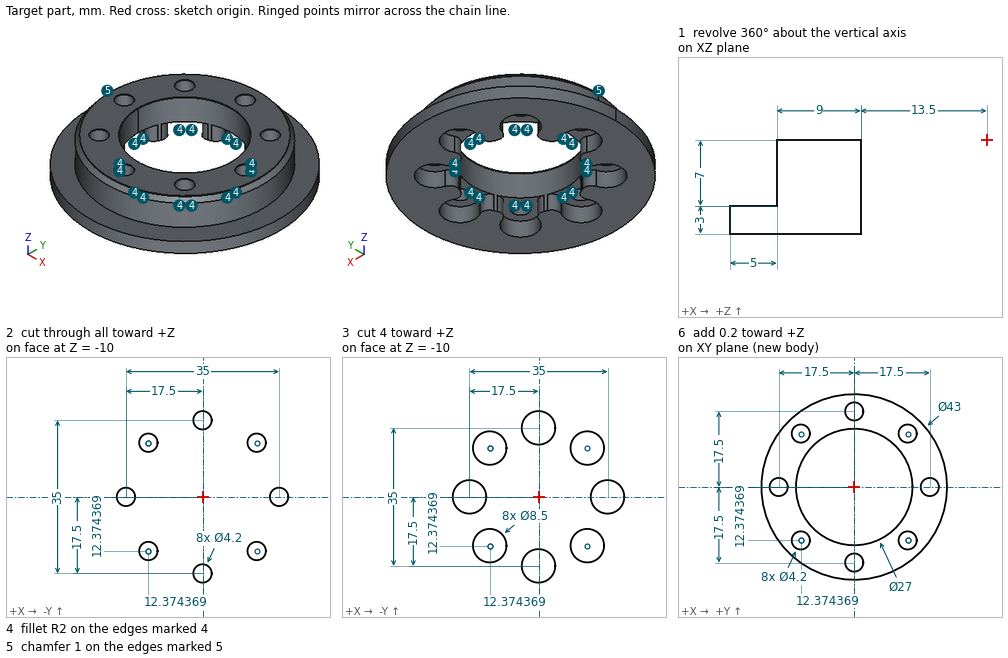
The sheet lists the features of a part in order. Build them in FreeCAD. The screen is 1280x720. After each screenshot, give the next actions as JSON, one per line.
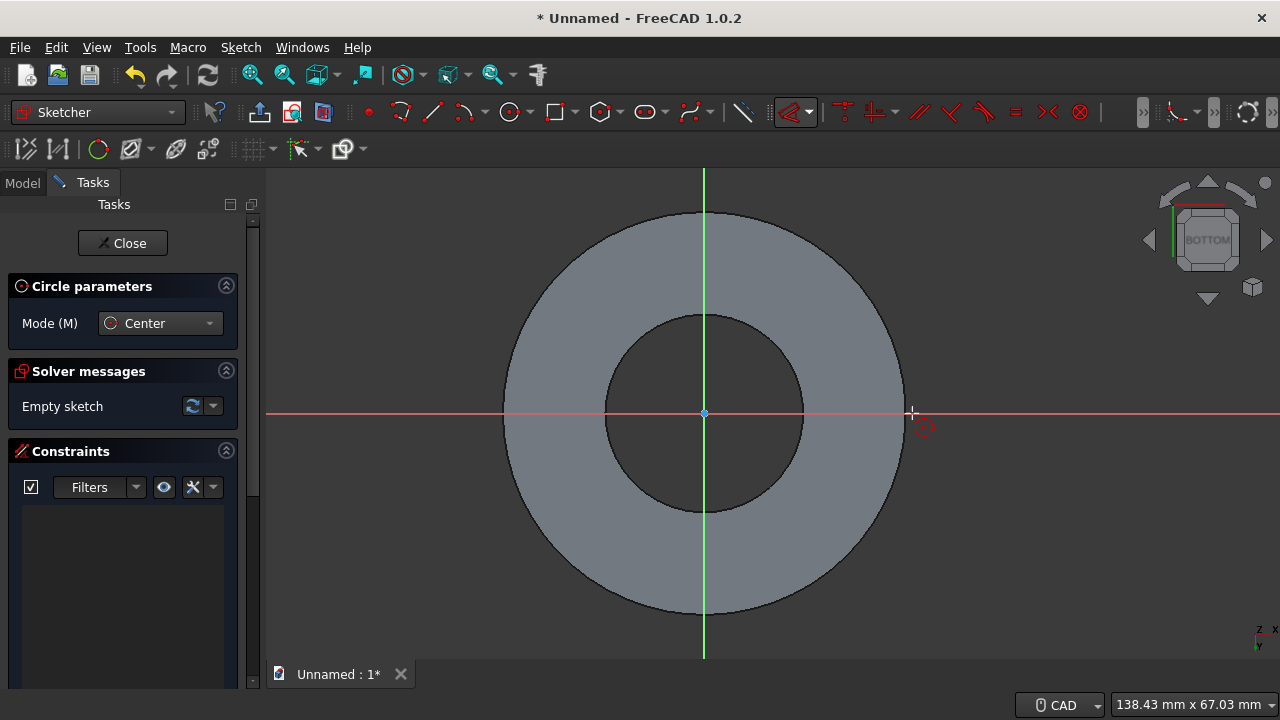
{"action": "scroll", "coordinate": [704, 542], "scroll_direction": "up", "scroll_amount": 2}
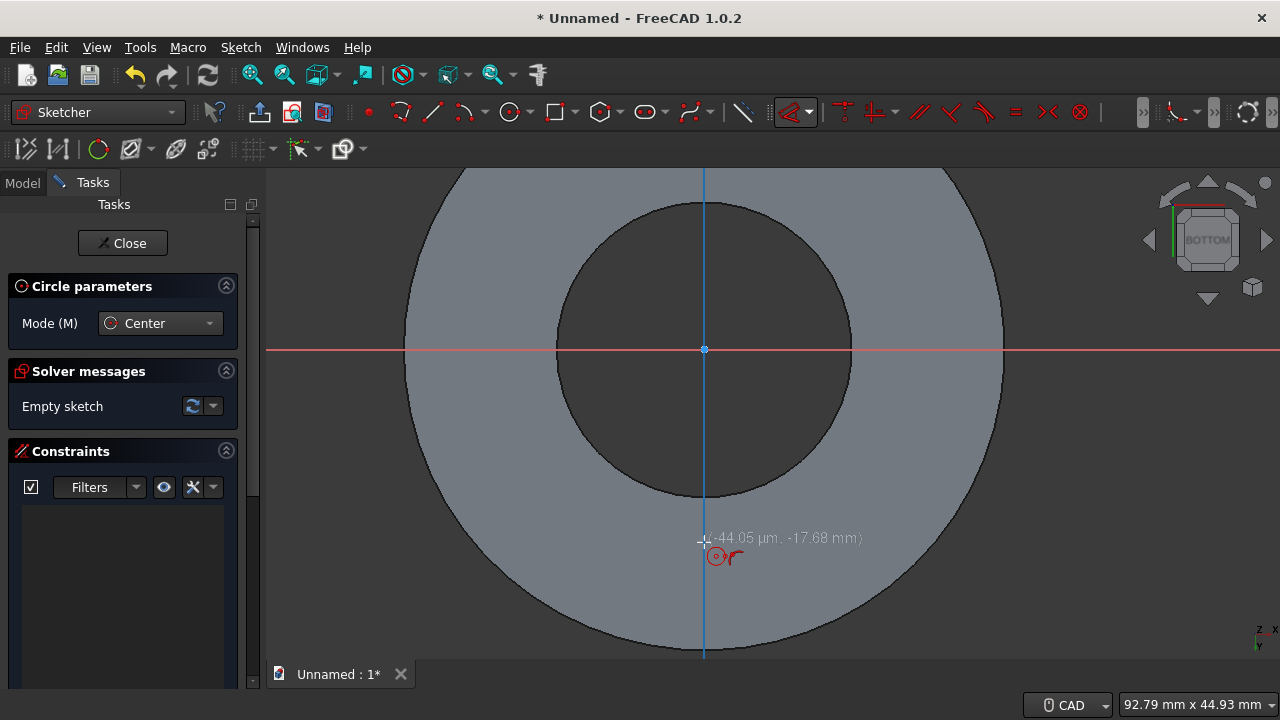
{"action": "left_click", "coordinate": [704, 541]}
{"action": "mouse_move", "coordinate": [720, 525]}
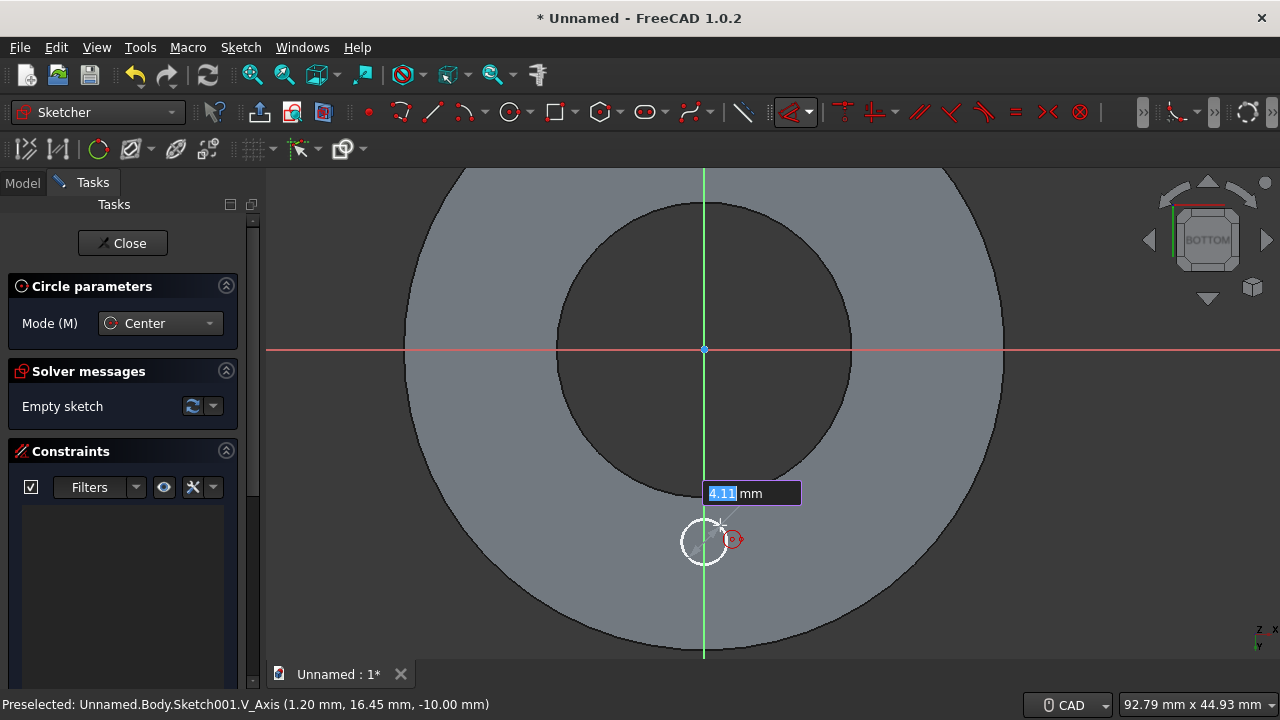
{"action": "type", "text": "4.2"}
{"action": "key", "text": "Return"}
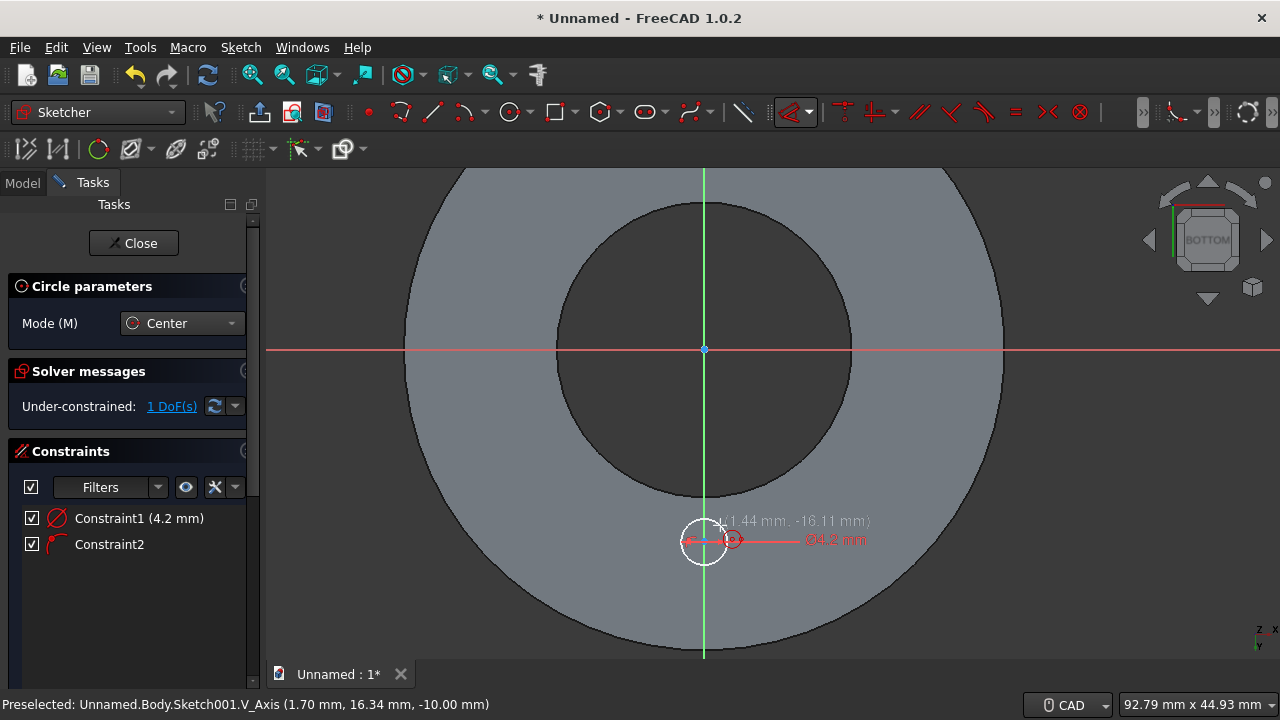
{"action": "left_click", "coordinate": [569, 485]}
{"action": "mouse_move", "coordinate": [585, 469]}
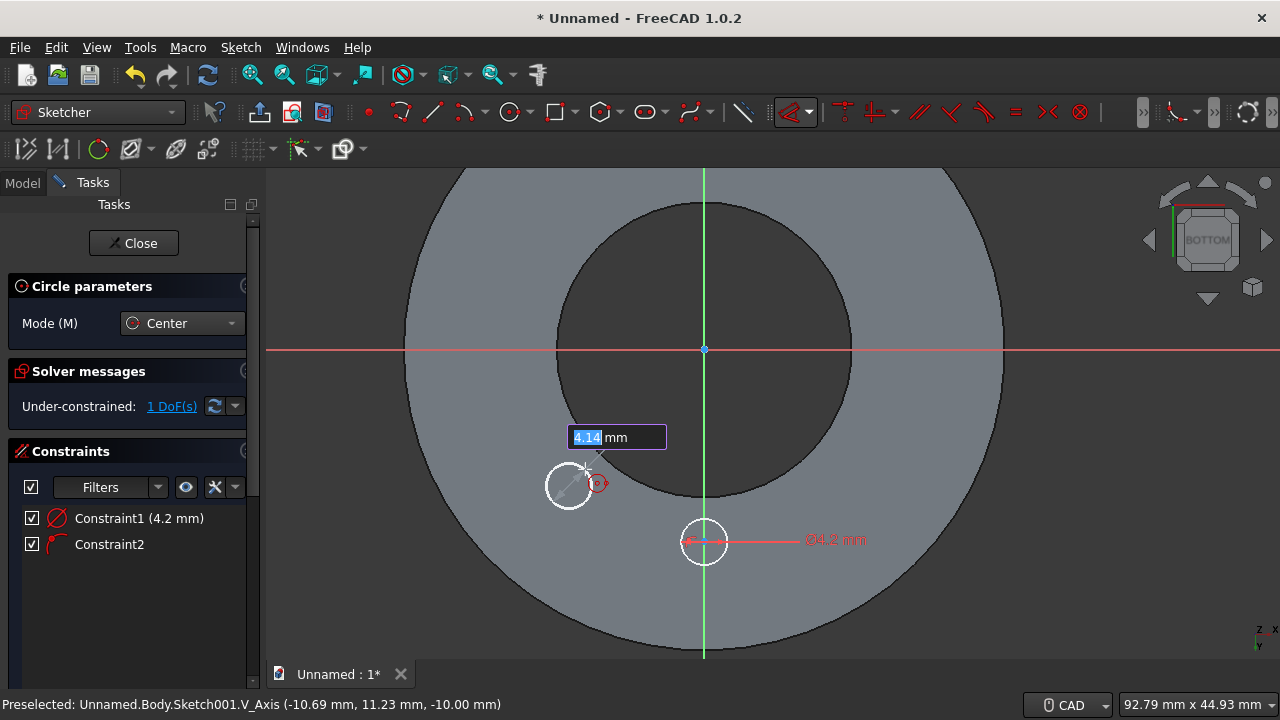
{"action": "type", "text": "4.2"}
{"action": "key", "text": "Return"}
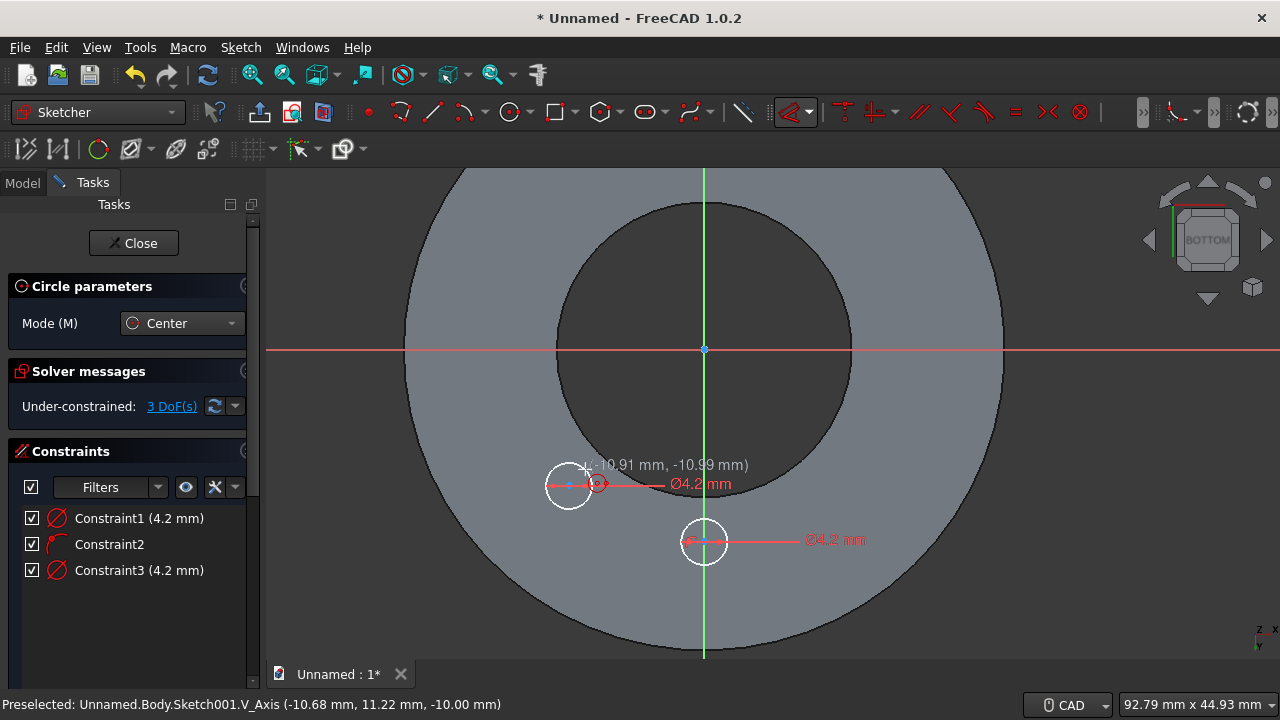
{"action": "left_click", "coordinate": [513, 350]}
{"action": "mouse_move", "coordinate": [529, 334]}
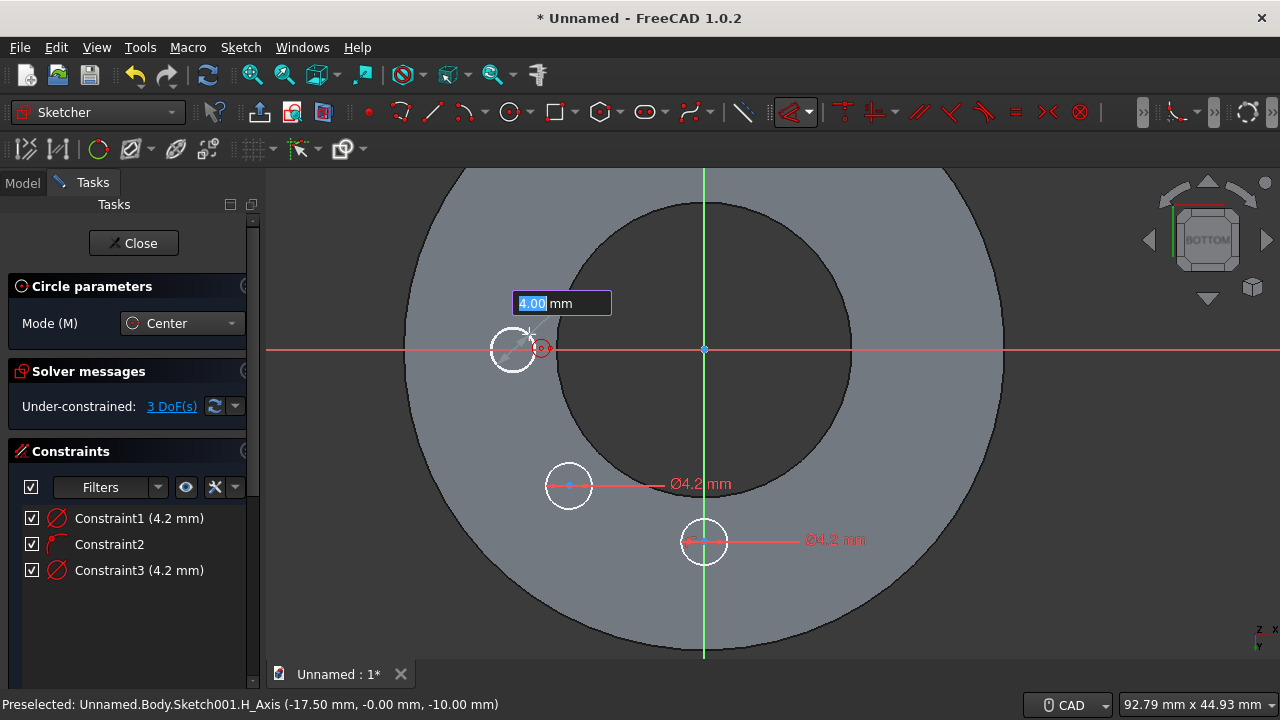
{"action": "type", "text": "4.2"}
{"action": "key", "text": "Return"}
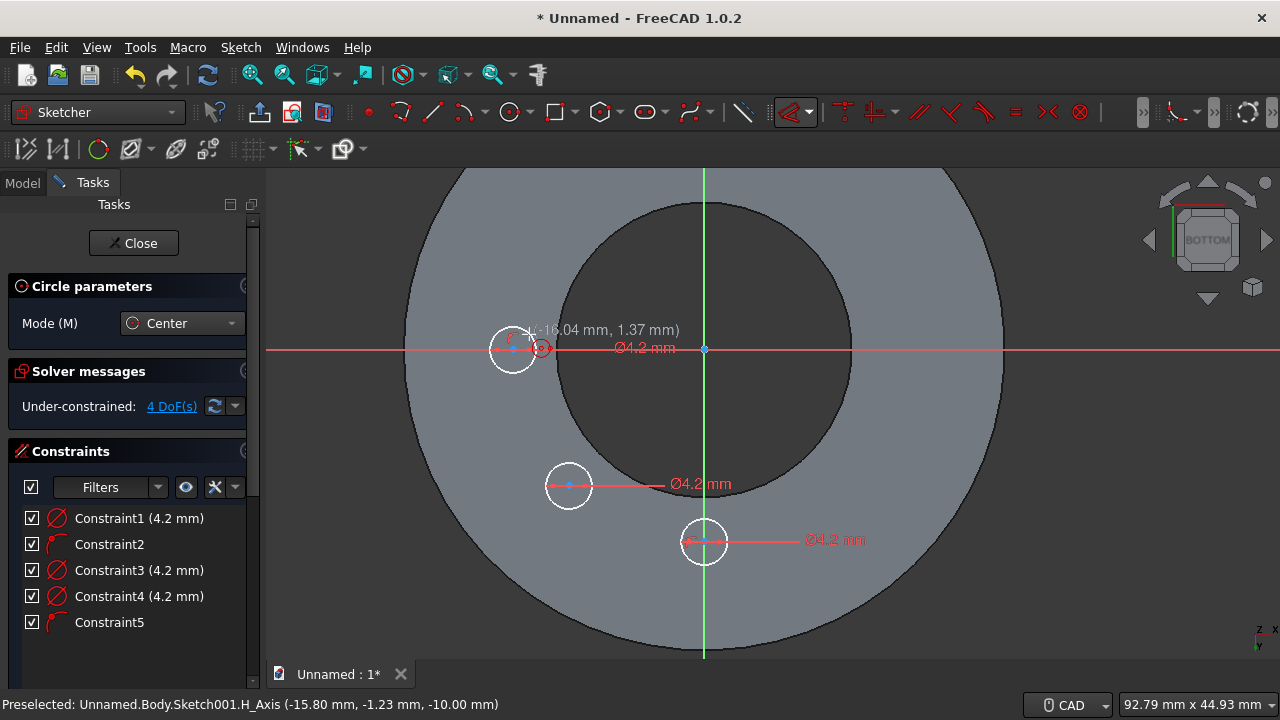
{"action": "left_click", "coordinate": [569, 215]}
{"action": "mouse_move", "coordinate": [585, 198]}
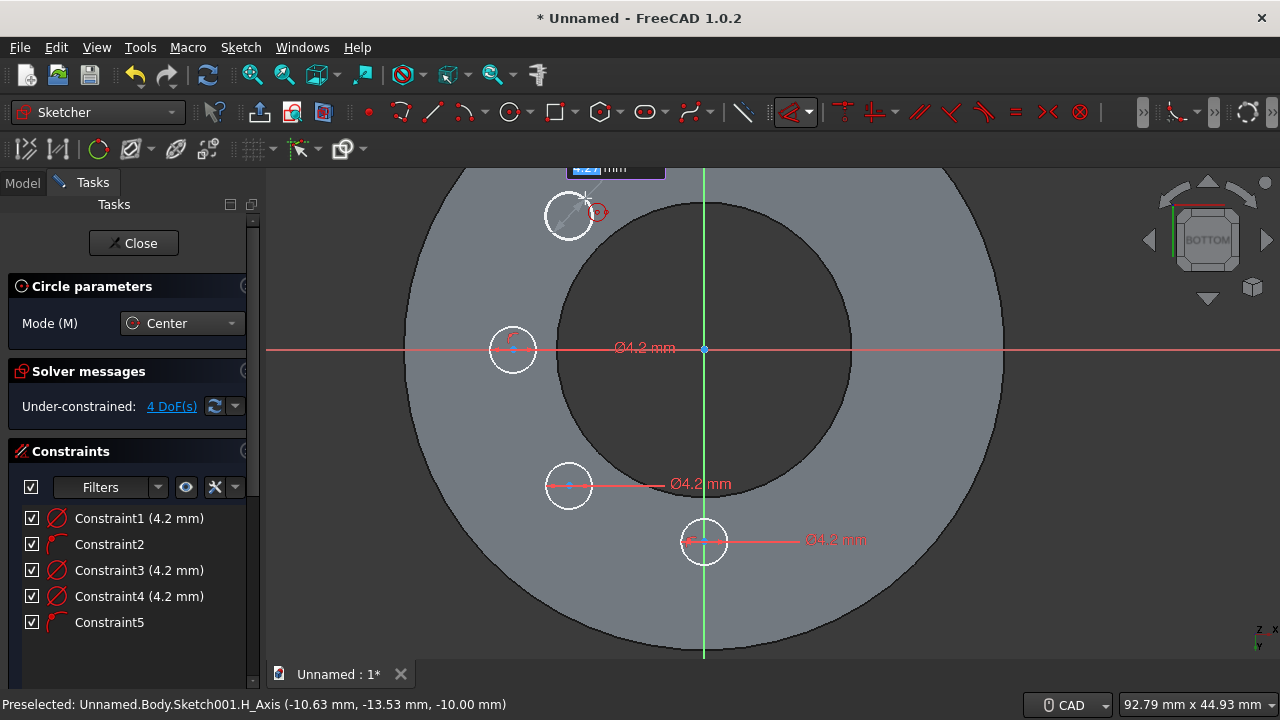
{"action": "type", "text": "4.2"}
{"action": "key", "text": "Return"}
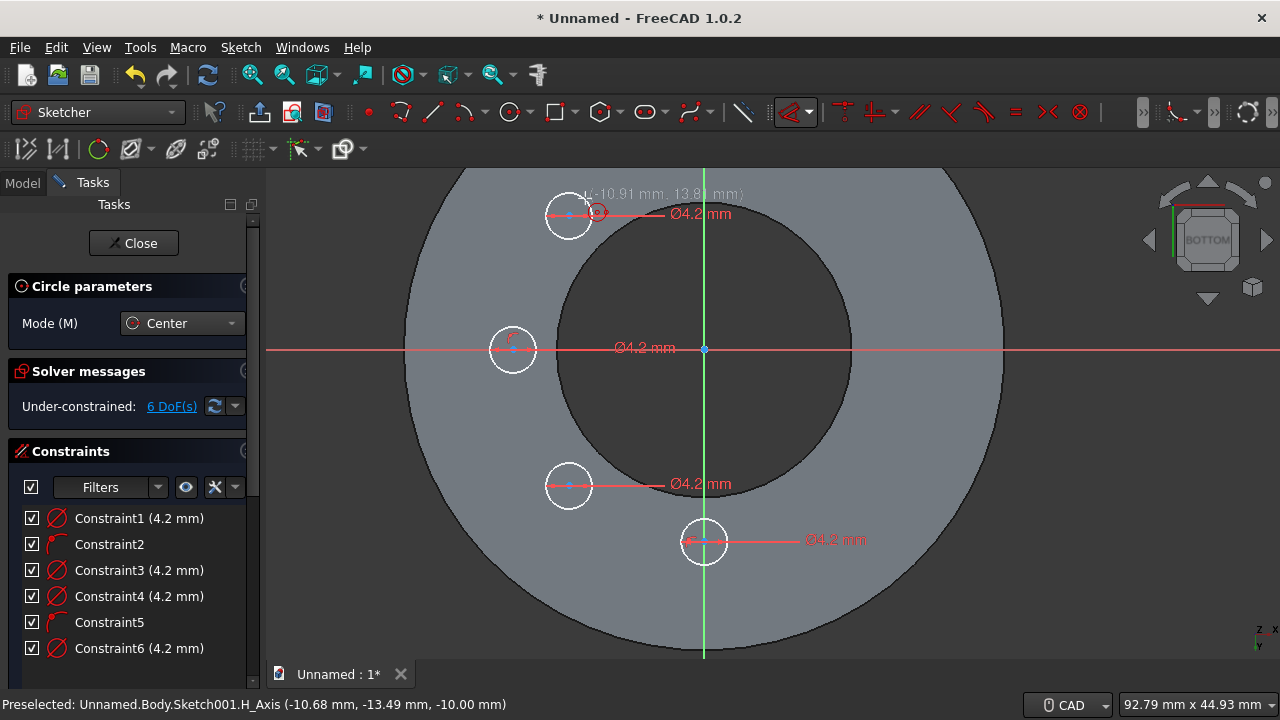
{"action": "scroll", "coordinate": [705, 543], "scroll_direction": "down", "scroll_amount": 2}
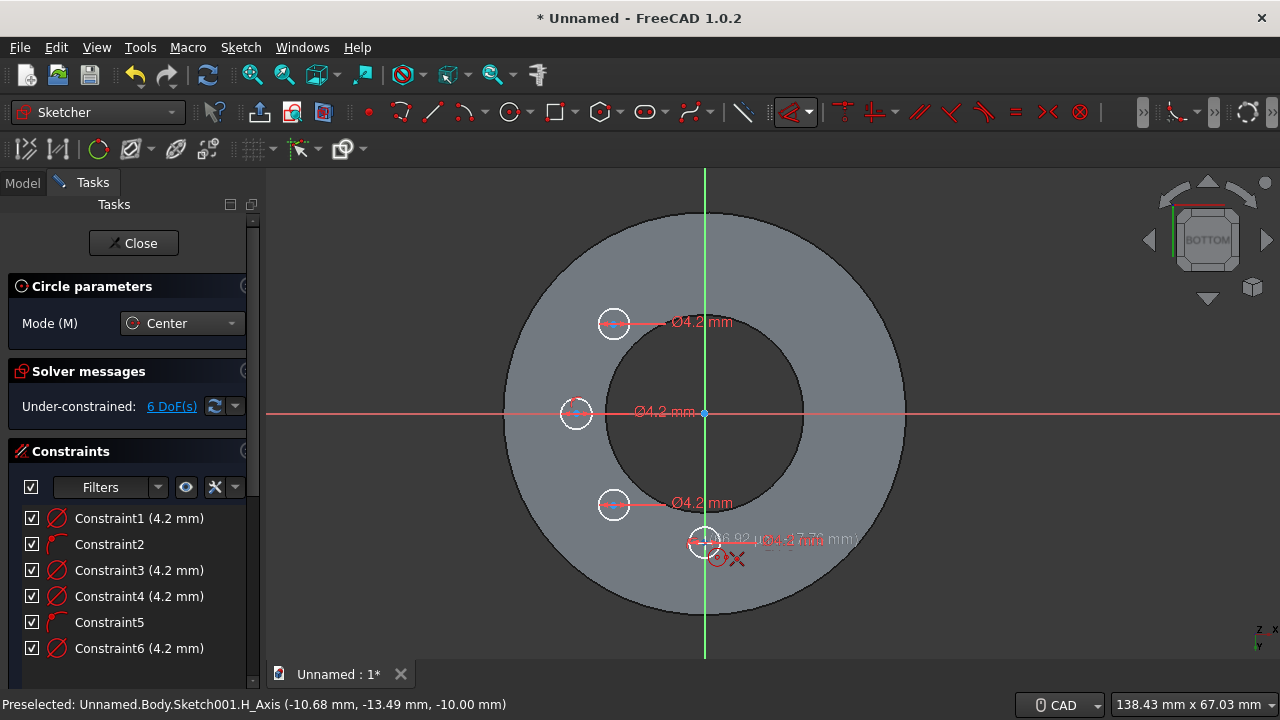
{"action": "scroll", "coordinate": [705, 286], "scroll_direction": "up", "scroll_amount": 2}